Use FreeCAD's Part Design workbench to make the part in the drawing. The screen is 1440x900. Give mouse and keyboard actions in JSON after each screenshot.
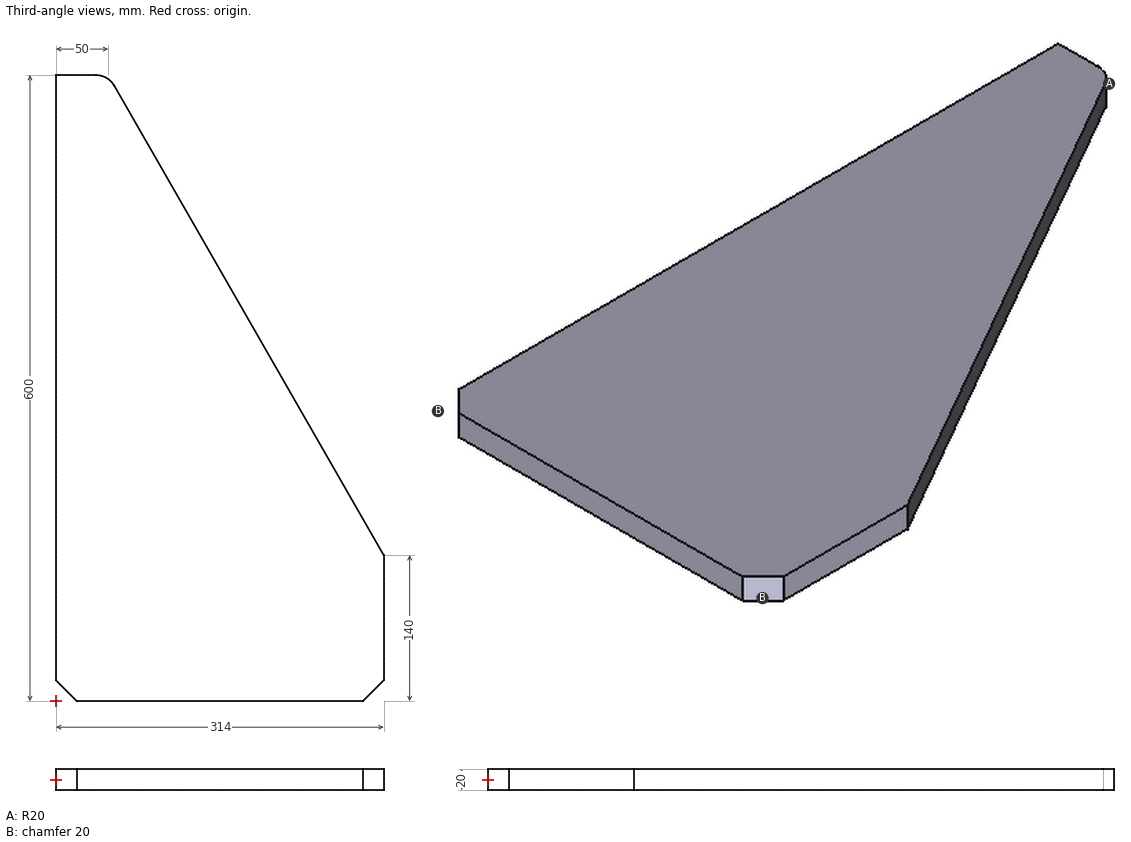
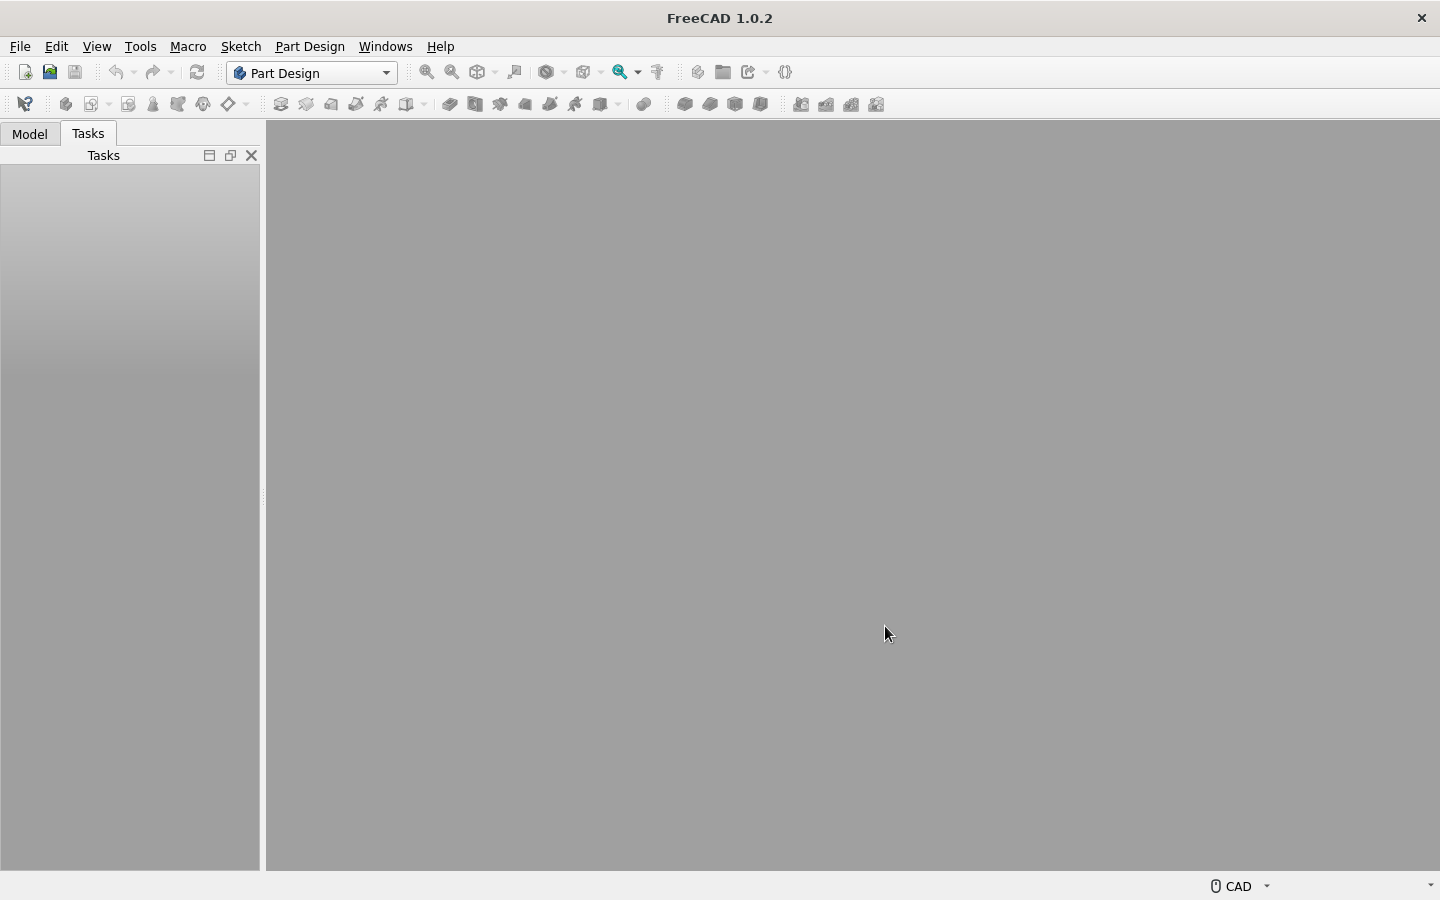
{"action": "left_click", "coordinate": [25, 72]}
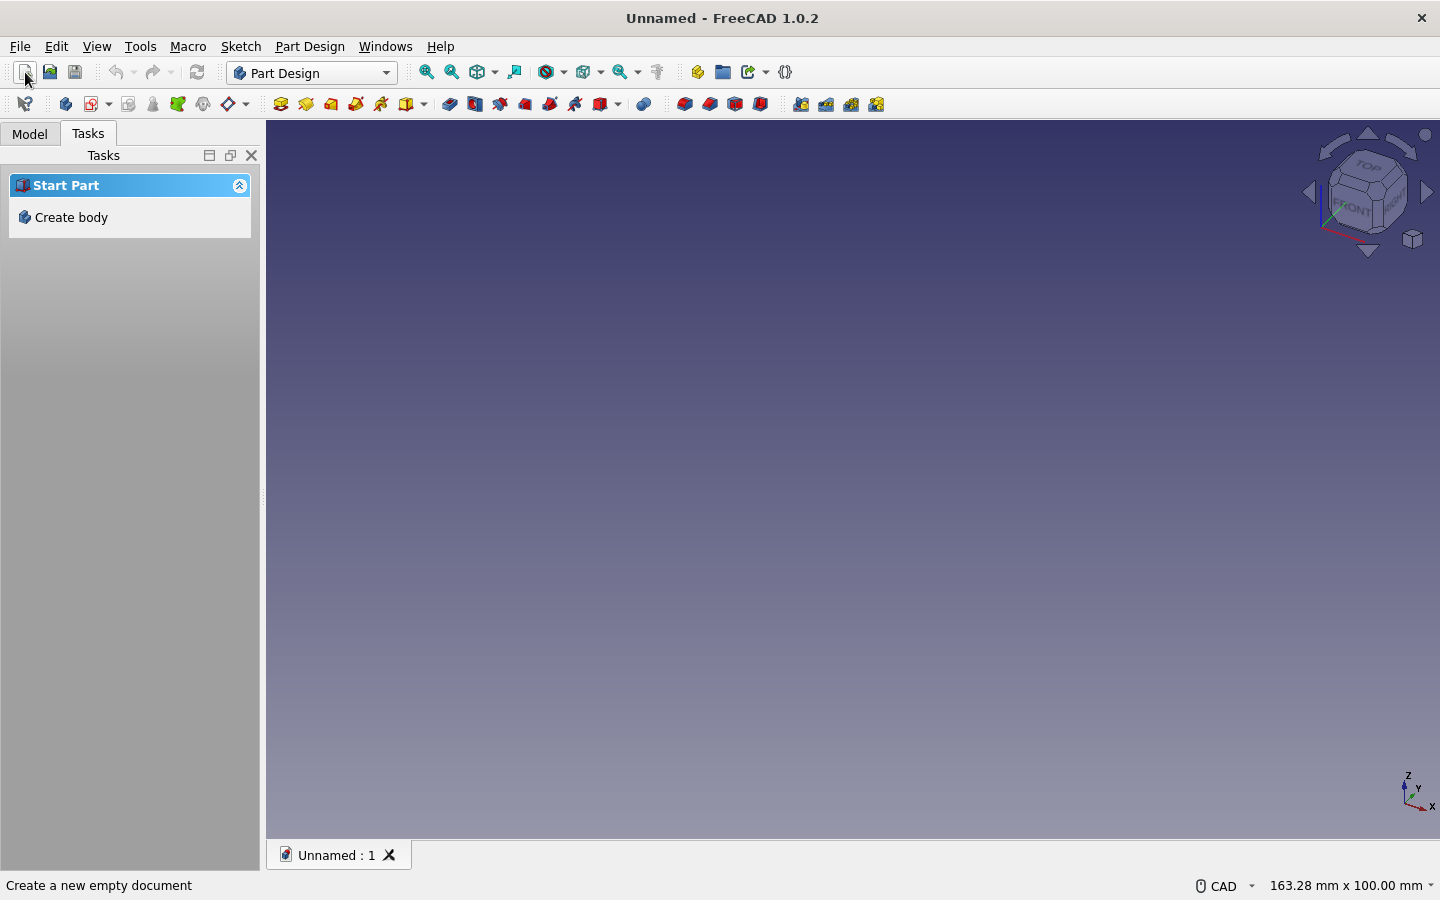
{"action": "left_click", "coordinate": [90, 104]}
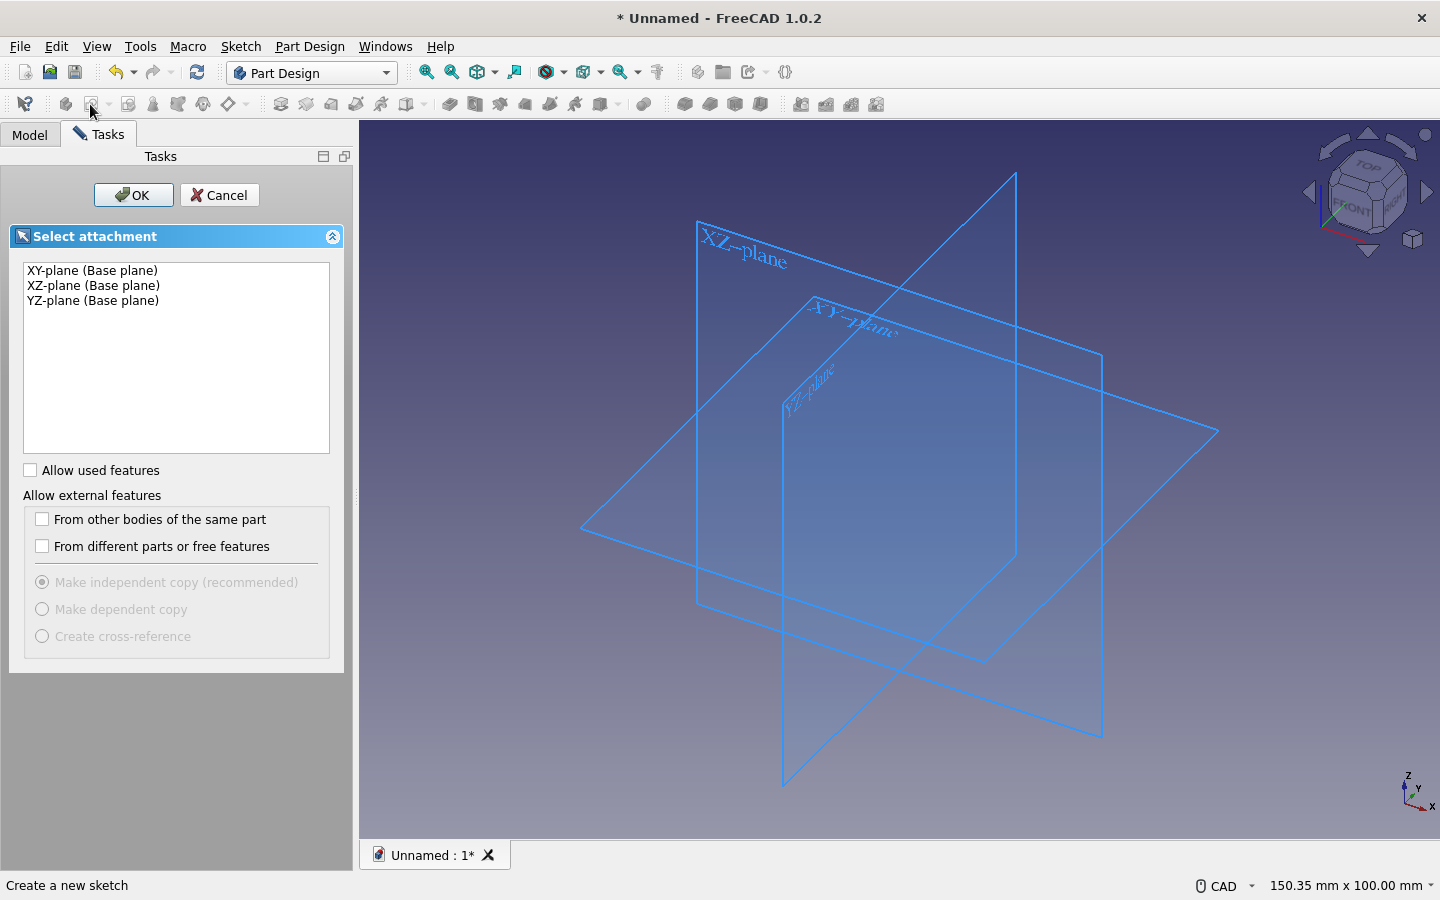
{"action": "left_click", "coordinate": [84, 270]}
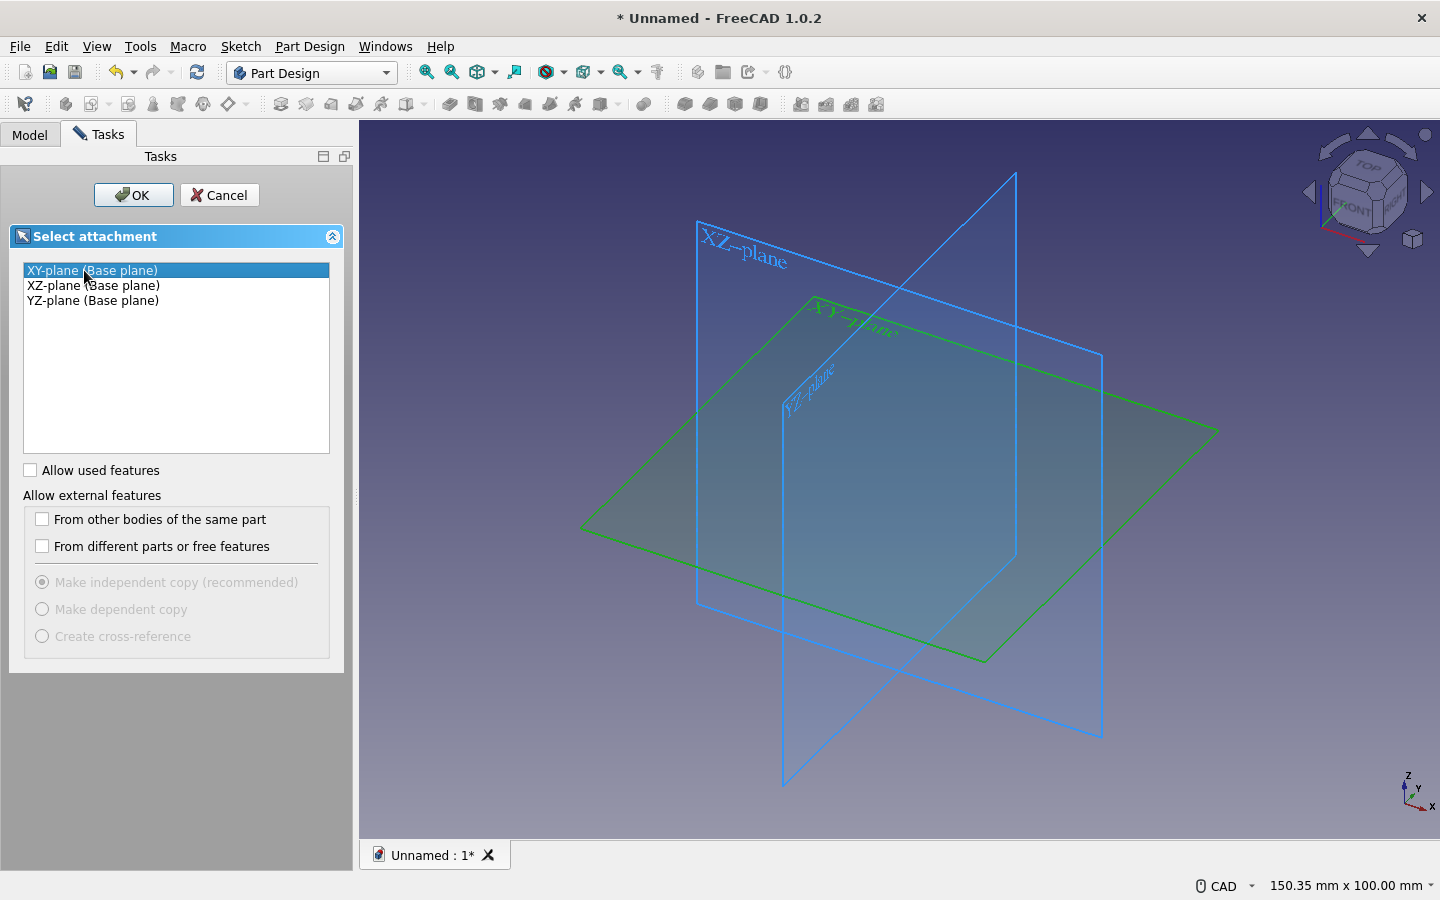
{"action": "left_click", "coordinate": [134, 195]}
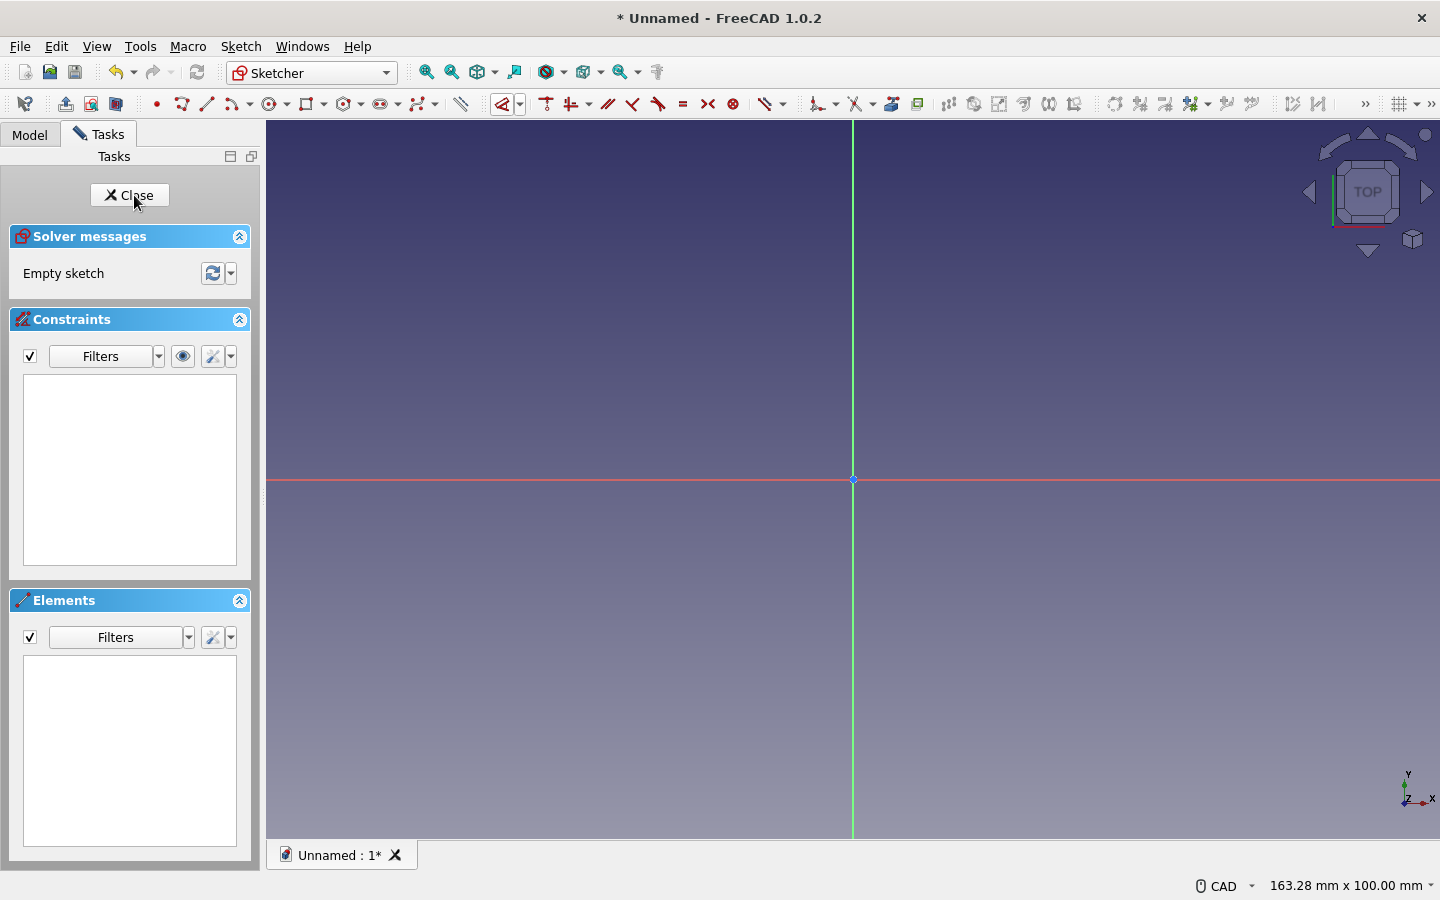
{"action": "scroll", "coordinate": [635, 748], "scroll_direction": "down", "scroll_amount": 11}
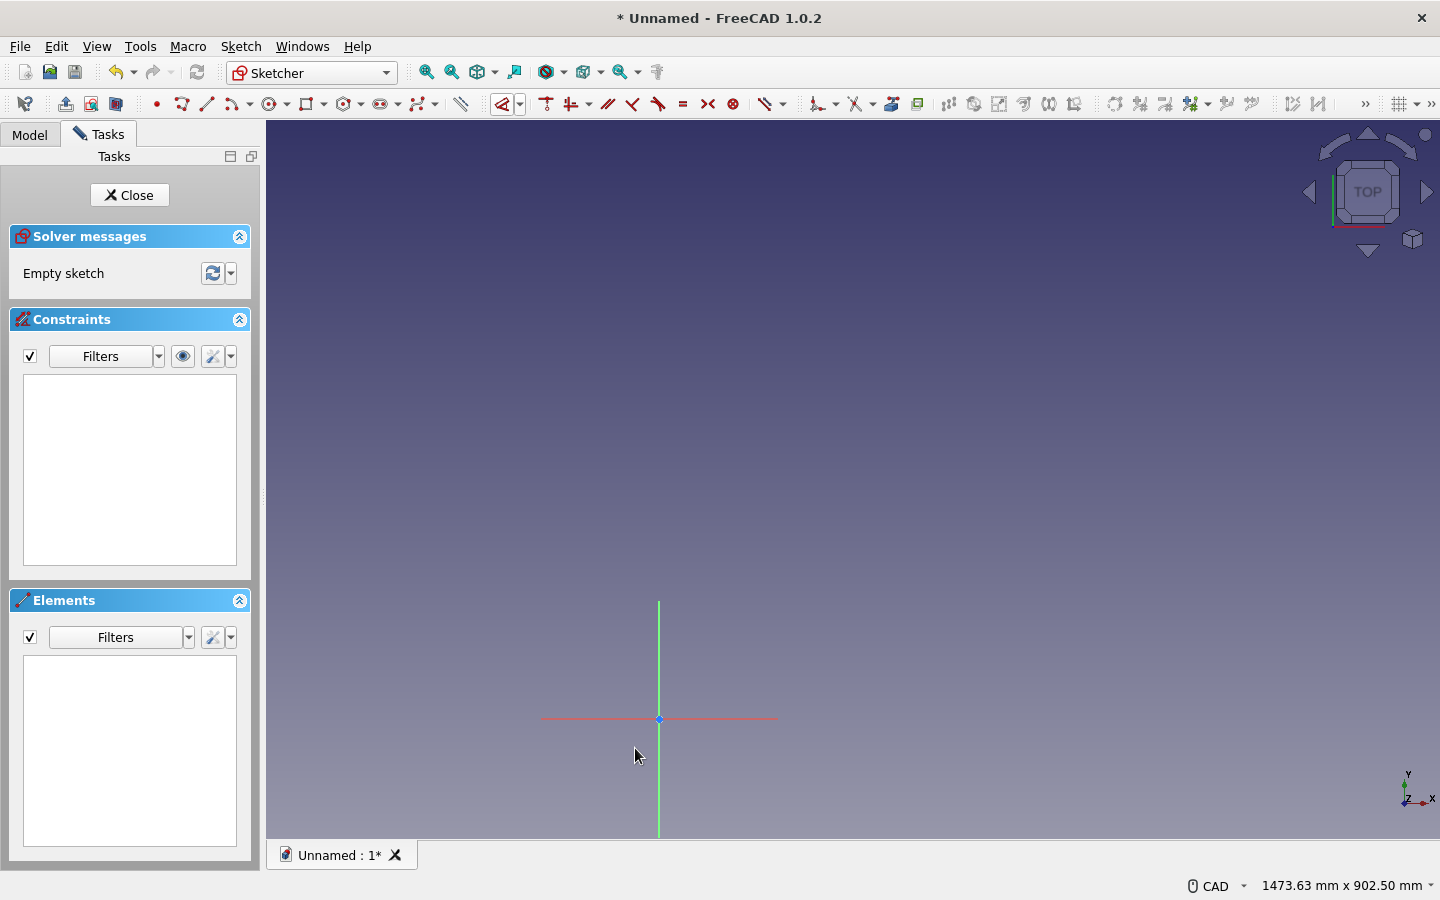
{"action": "left_click", "coordinate": [182, 104]}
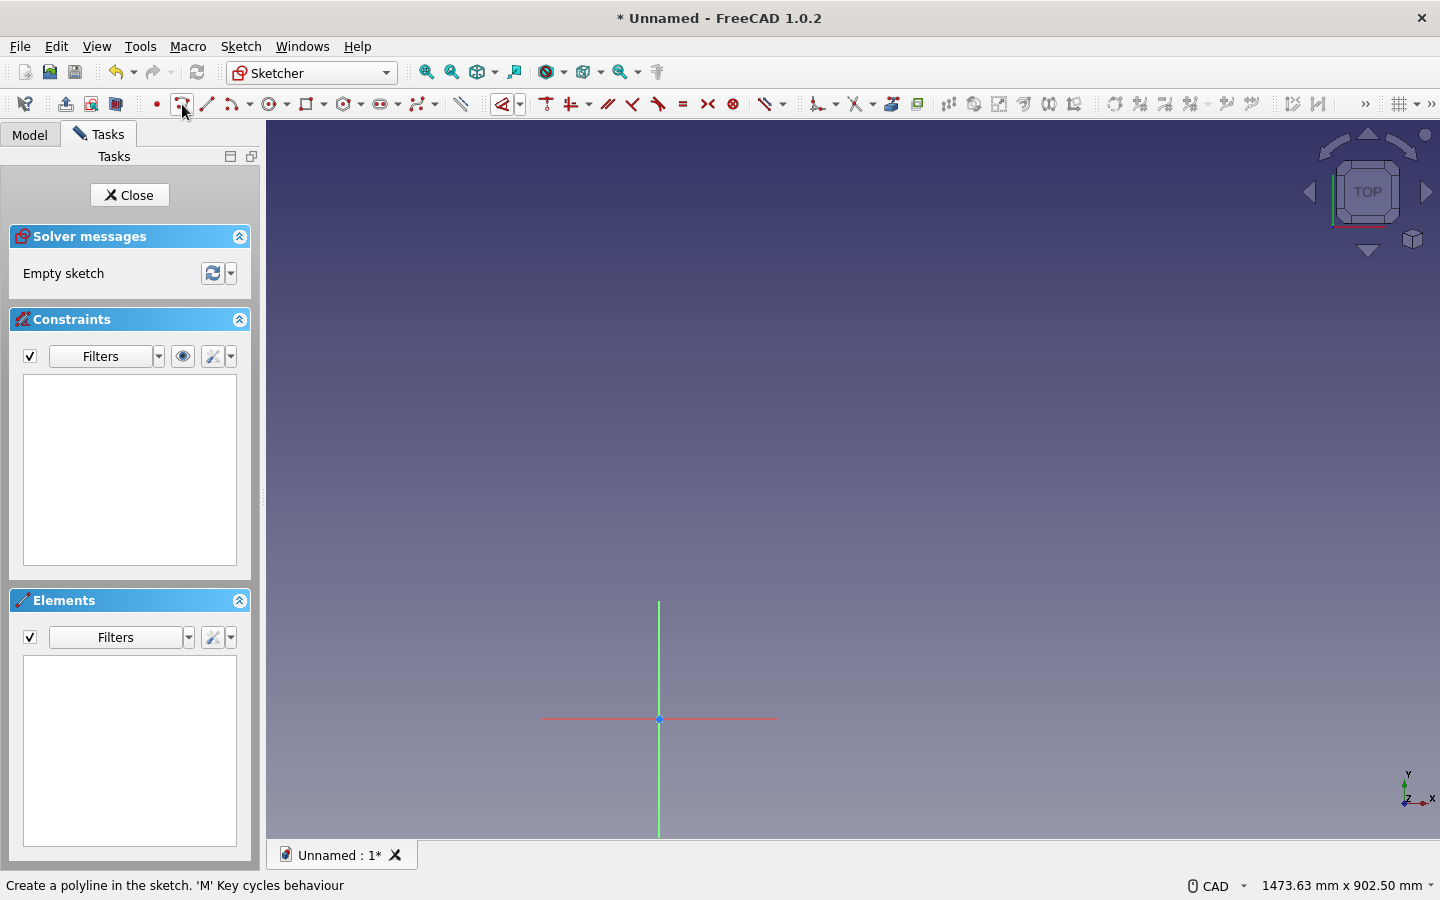
{"action": "left_click", "coordinate": [659, 719]}
{"action": "left_click", "coordinate": [910, 710]}
{"action": "left_click", "coordinate": [910, 607]}
{"action": "left_click", "coordinate": [699, 241]}
{"action": "left_click", "coordinate": [668, 241]}
{"action": "left_click", "coordinate": [659, 719]}
{"action": "key", "text": "Escape"}
{"action": "key", "text": "Escape"}